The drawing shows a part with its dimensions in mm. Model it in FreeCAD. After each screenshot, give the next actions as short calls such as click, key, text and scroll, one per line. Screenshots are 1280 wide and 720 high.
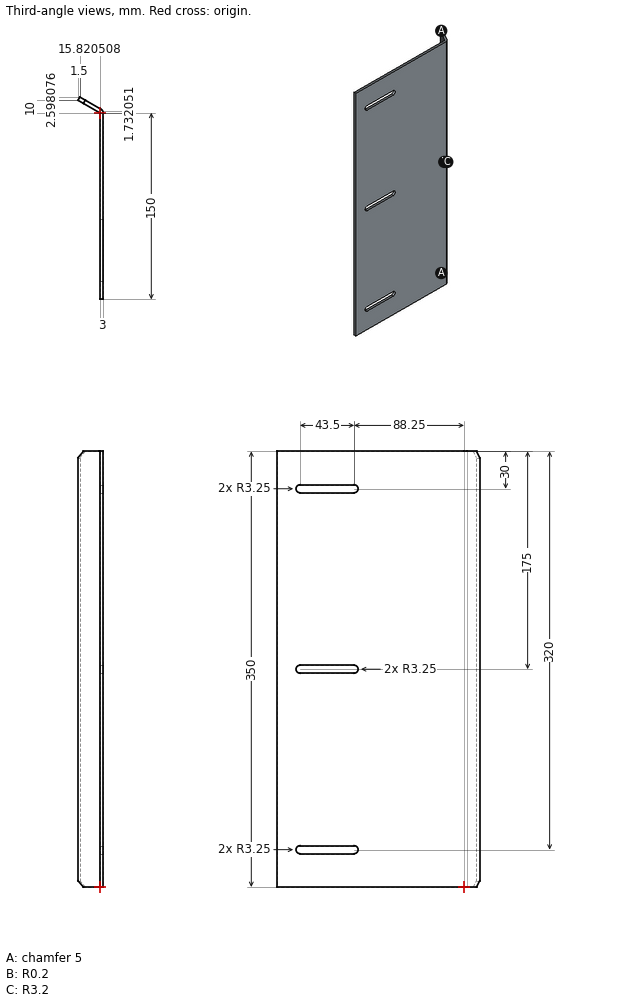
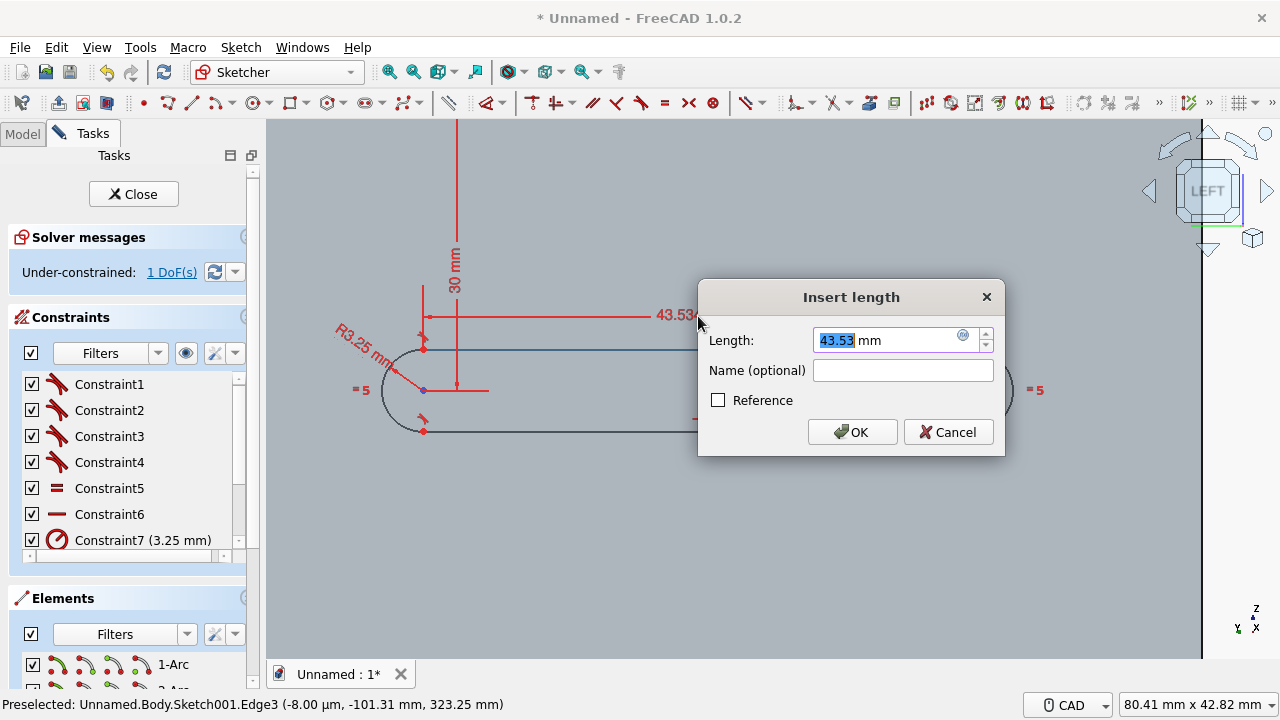
text(43.5)
key(Return)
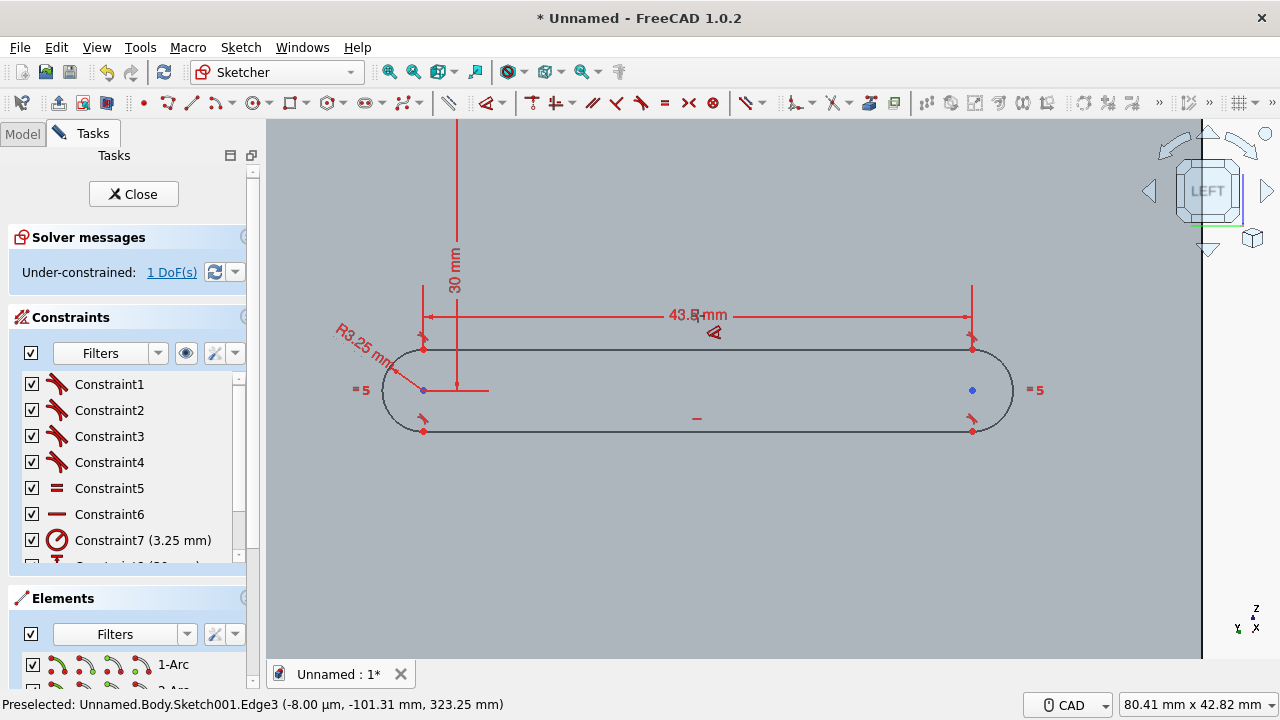
click(423, 350)
click(359, 384)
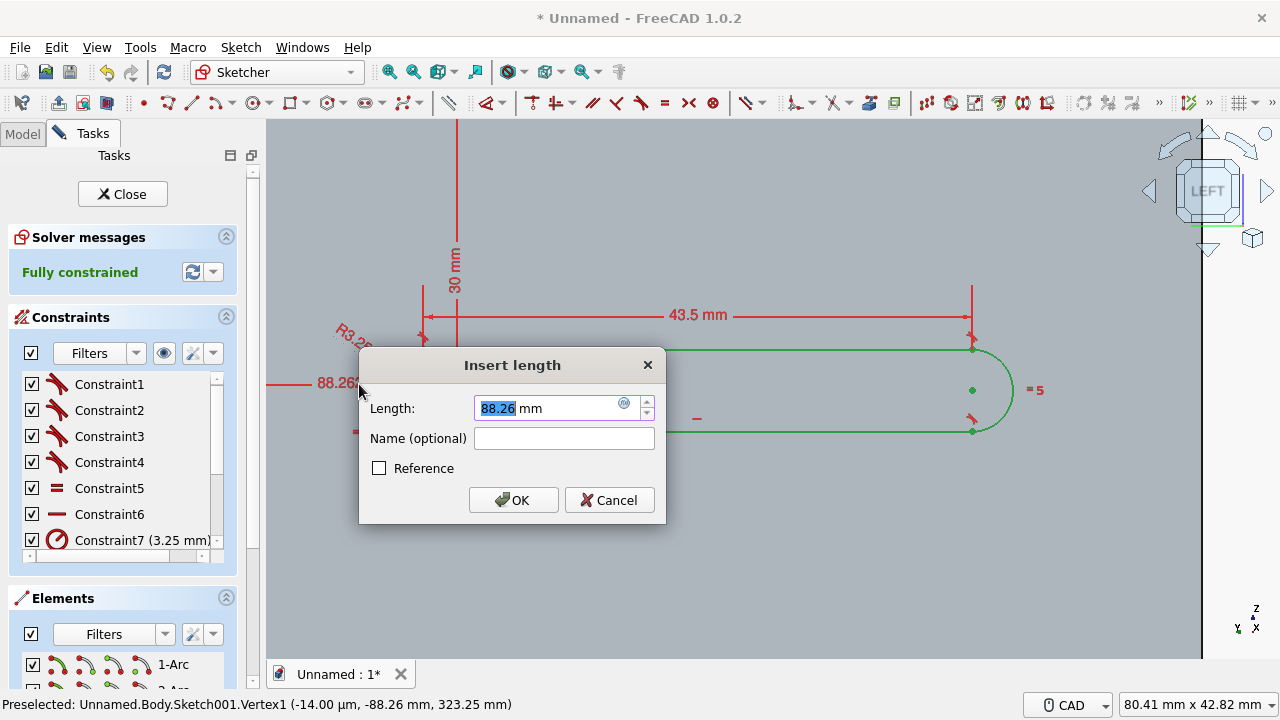
text(88.25)
key(Return)
key(Escape)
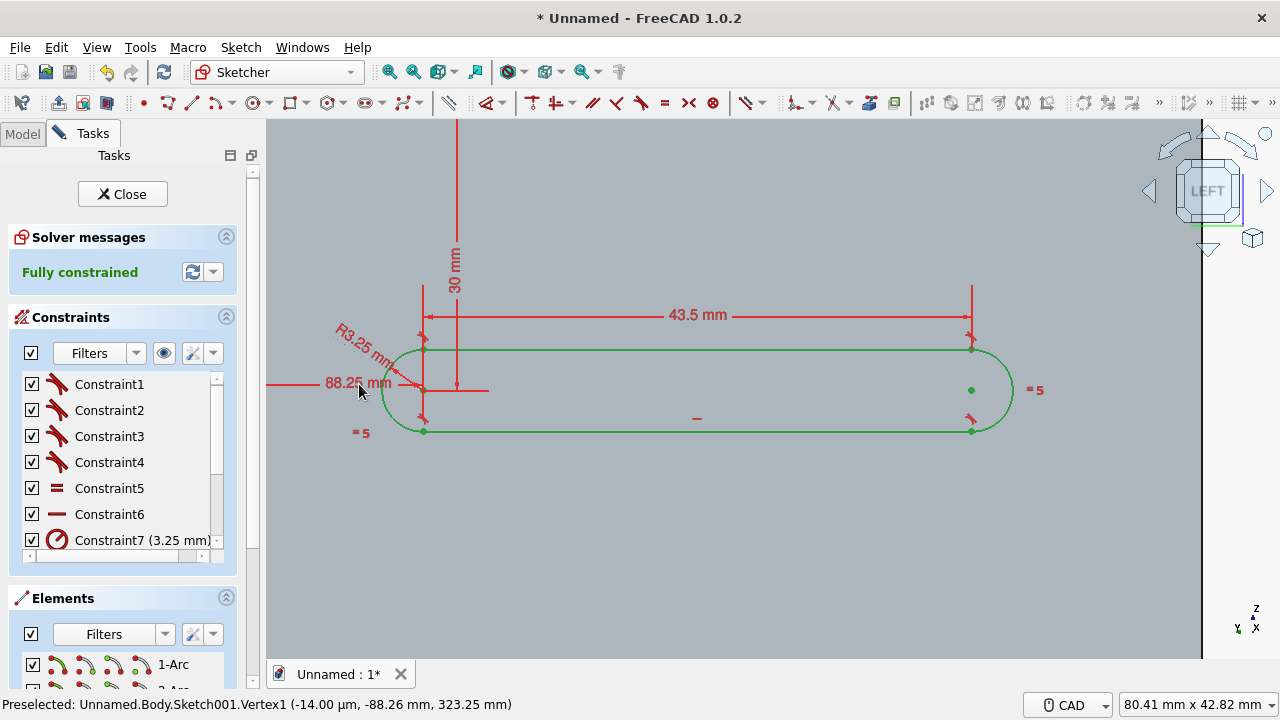
click(123, 194)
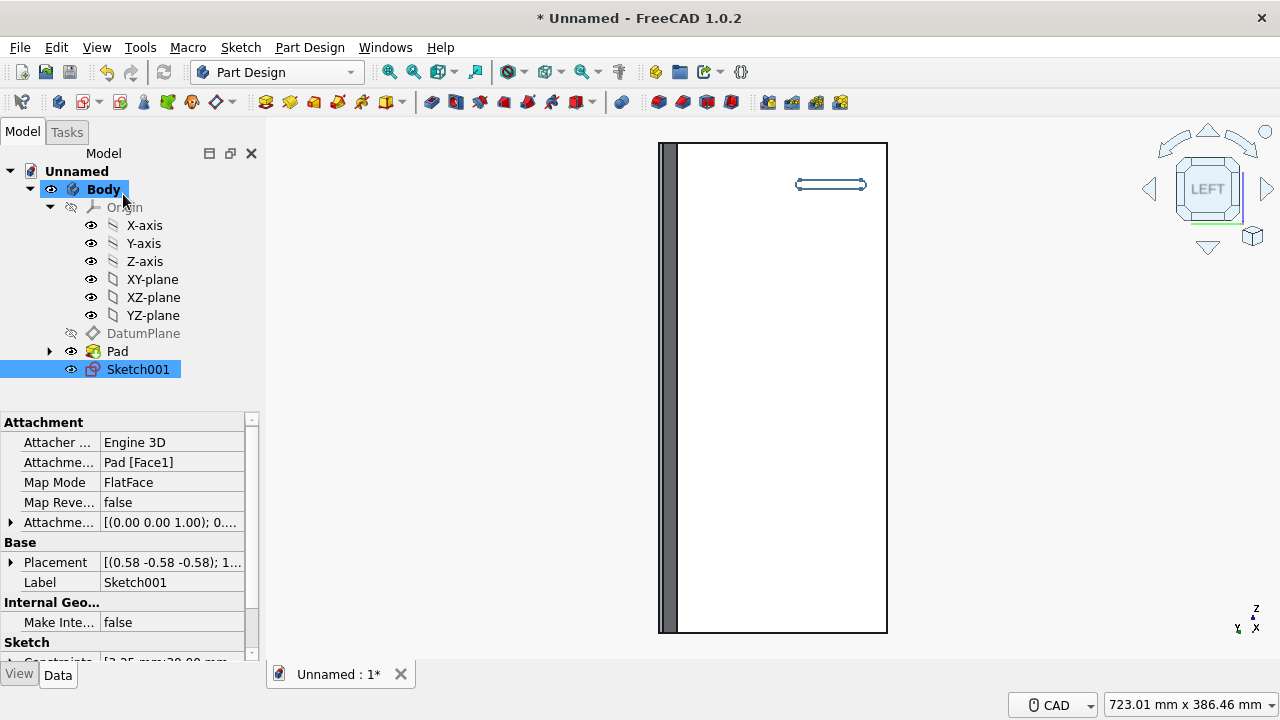
click(432, 102)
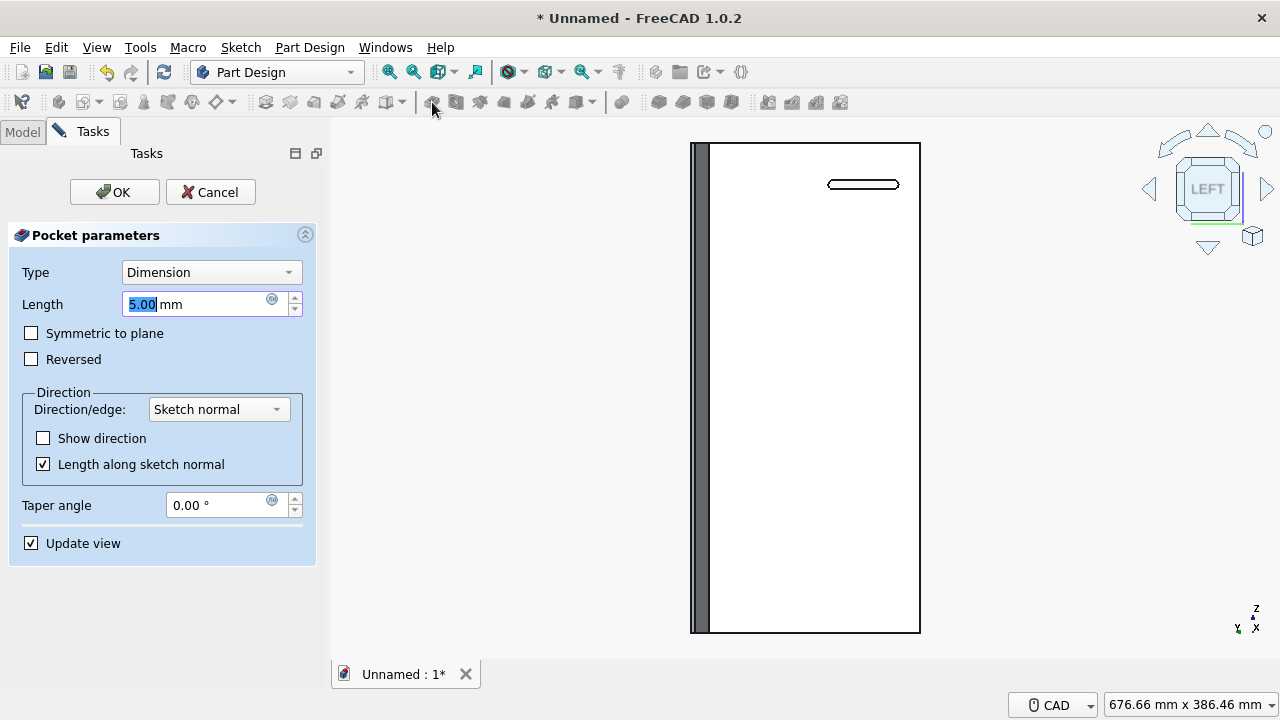
click(212, 272)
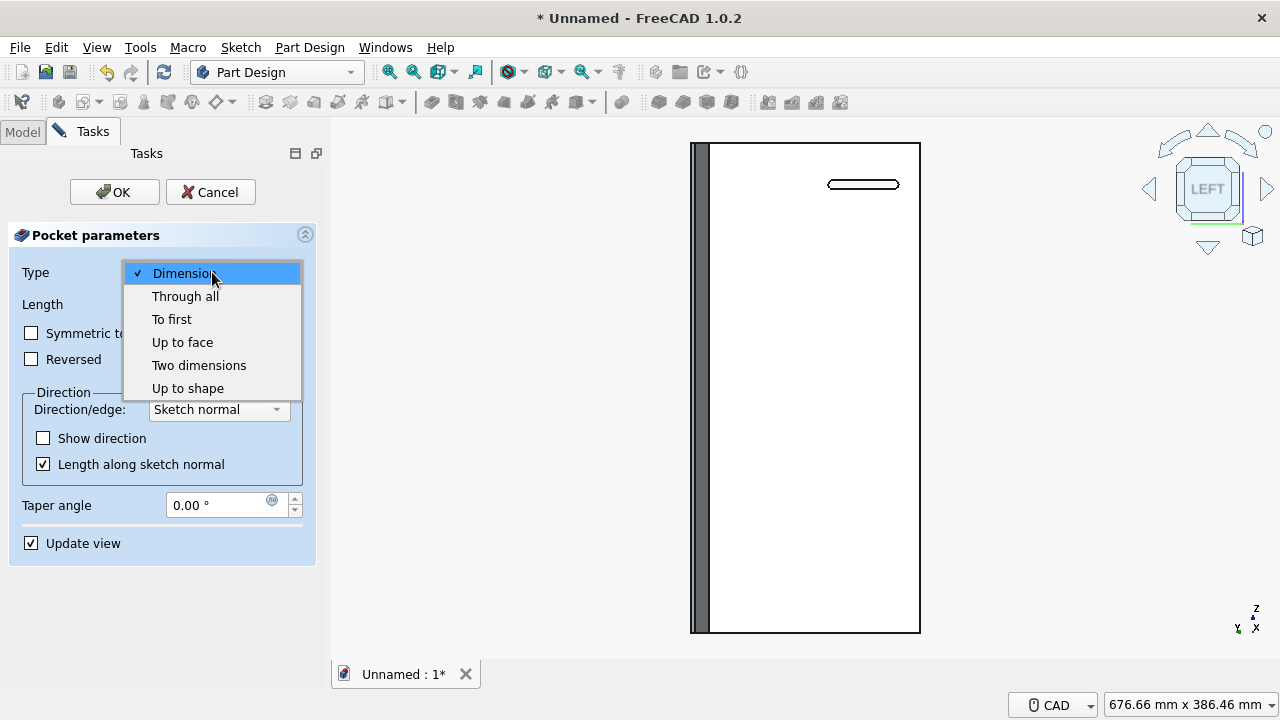
click(212, 296)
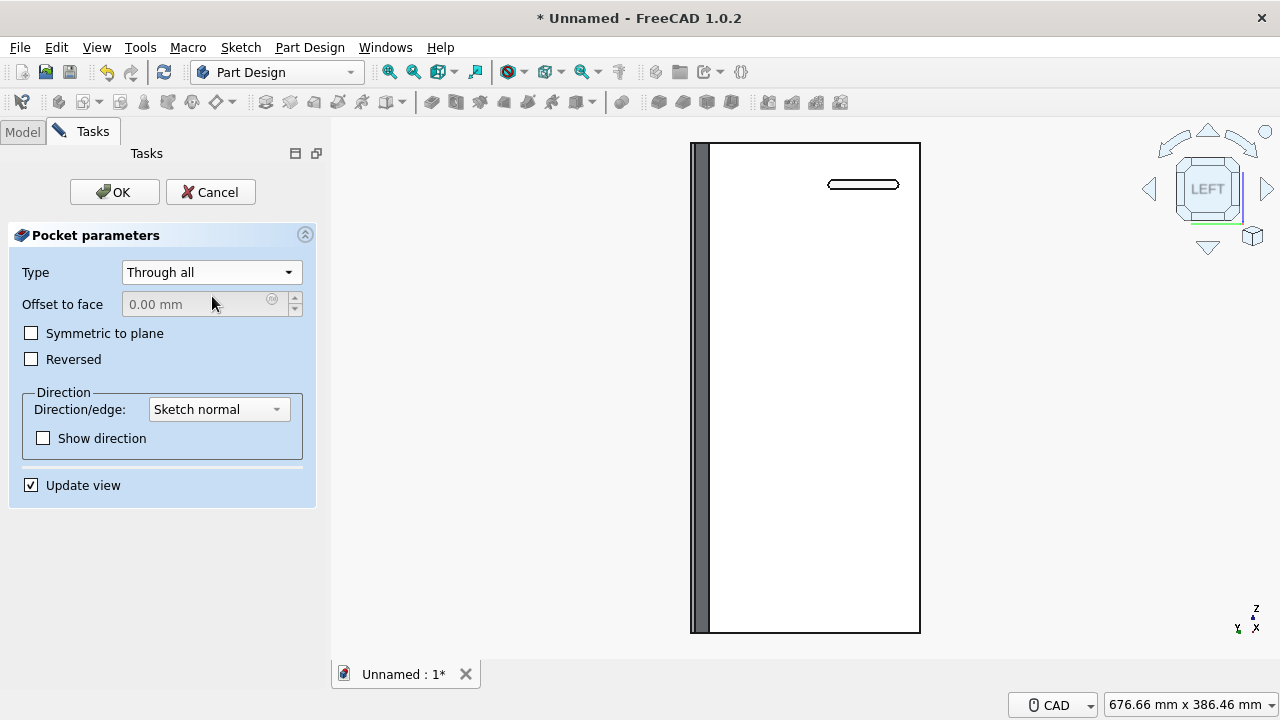
click(115, 192)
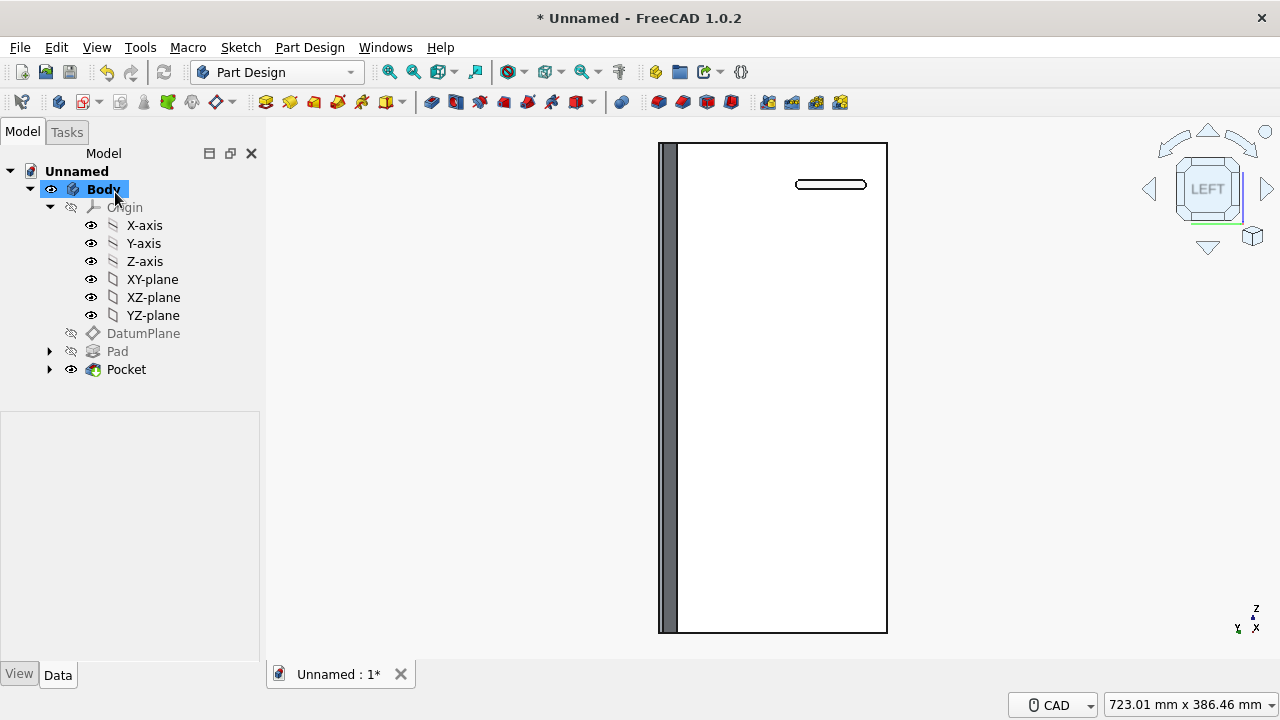
click(782, 317)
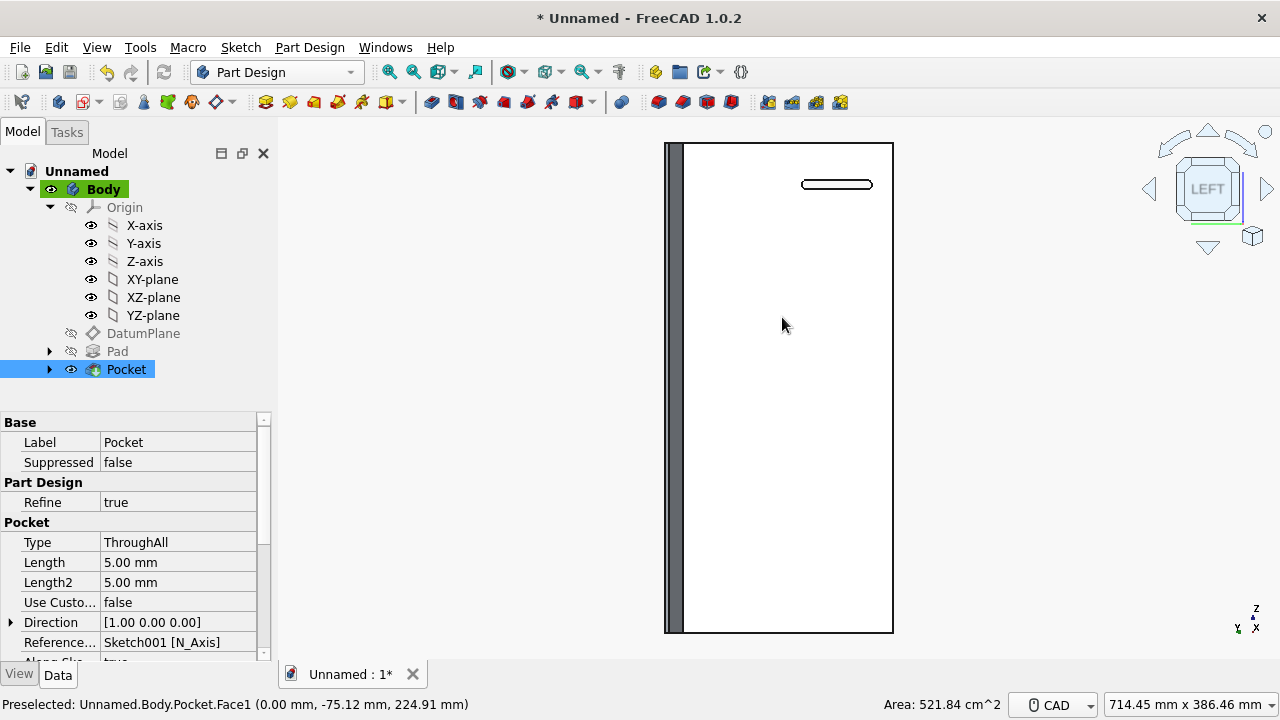
click(84, 102)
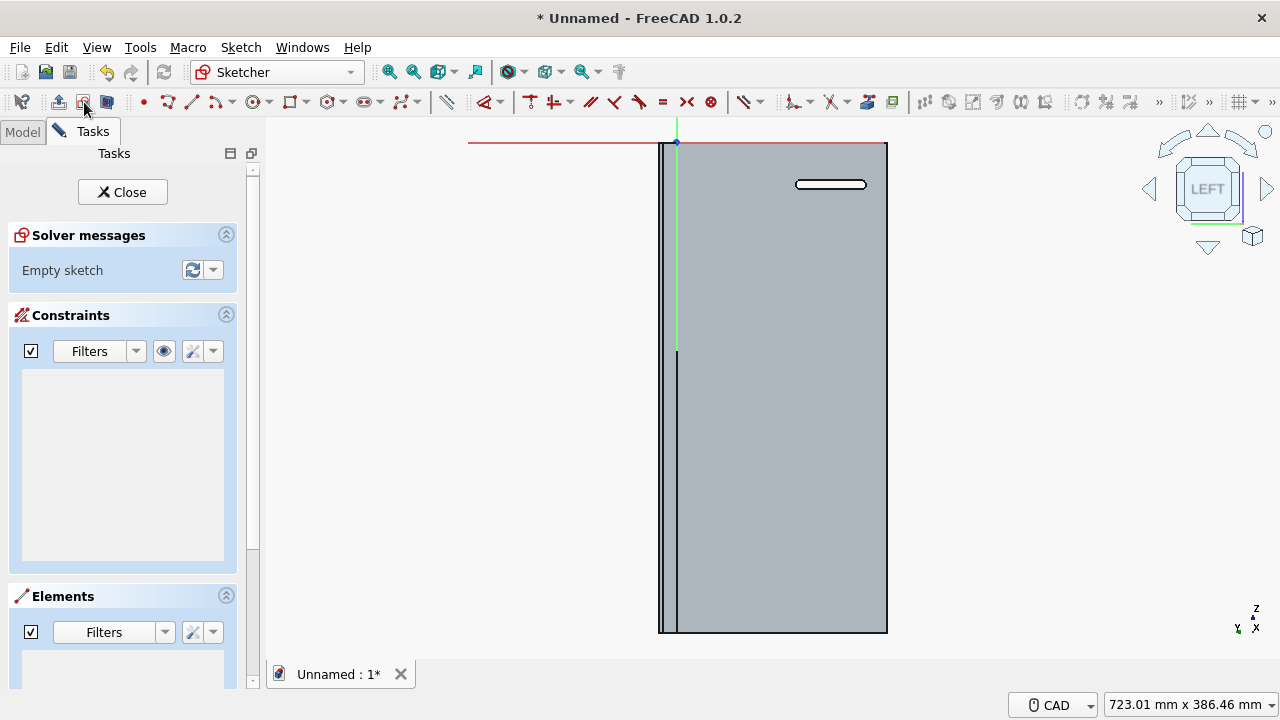
scroll(847, 617, up, 11)